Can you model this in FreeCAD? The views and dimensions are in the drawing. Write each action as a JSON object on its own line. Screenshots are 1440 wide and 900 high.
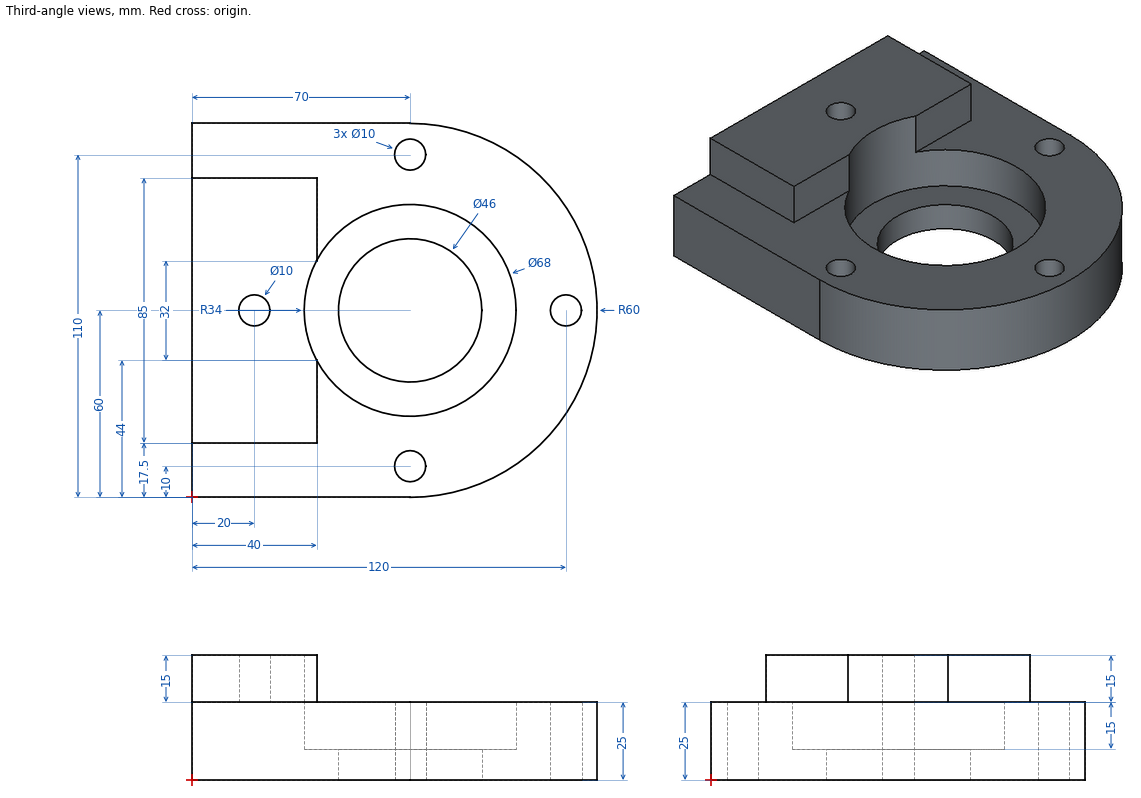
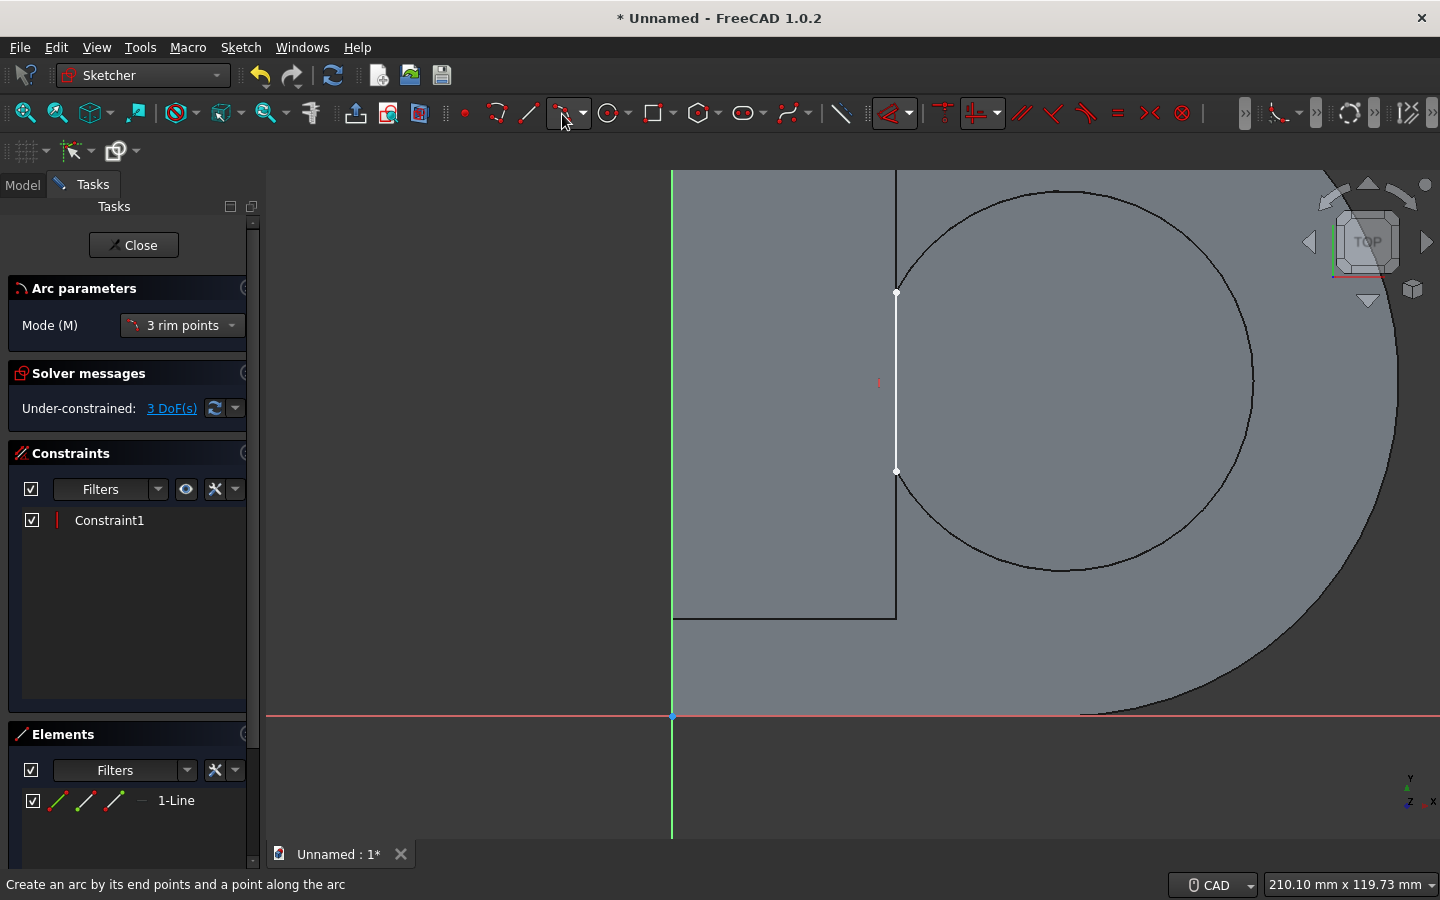
{"action": "left_click", "coordinate": [896, 293]}
{"action": "left_click", "coordinate": [896, 472]}
{"action": "left_click", "coordinate": [874, 381]}
{"action": "key", "text": "Escape"}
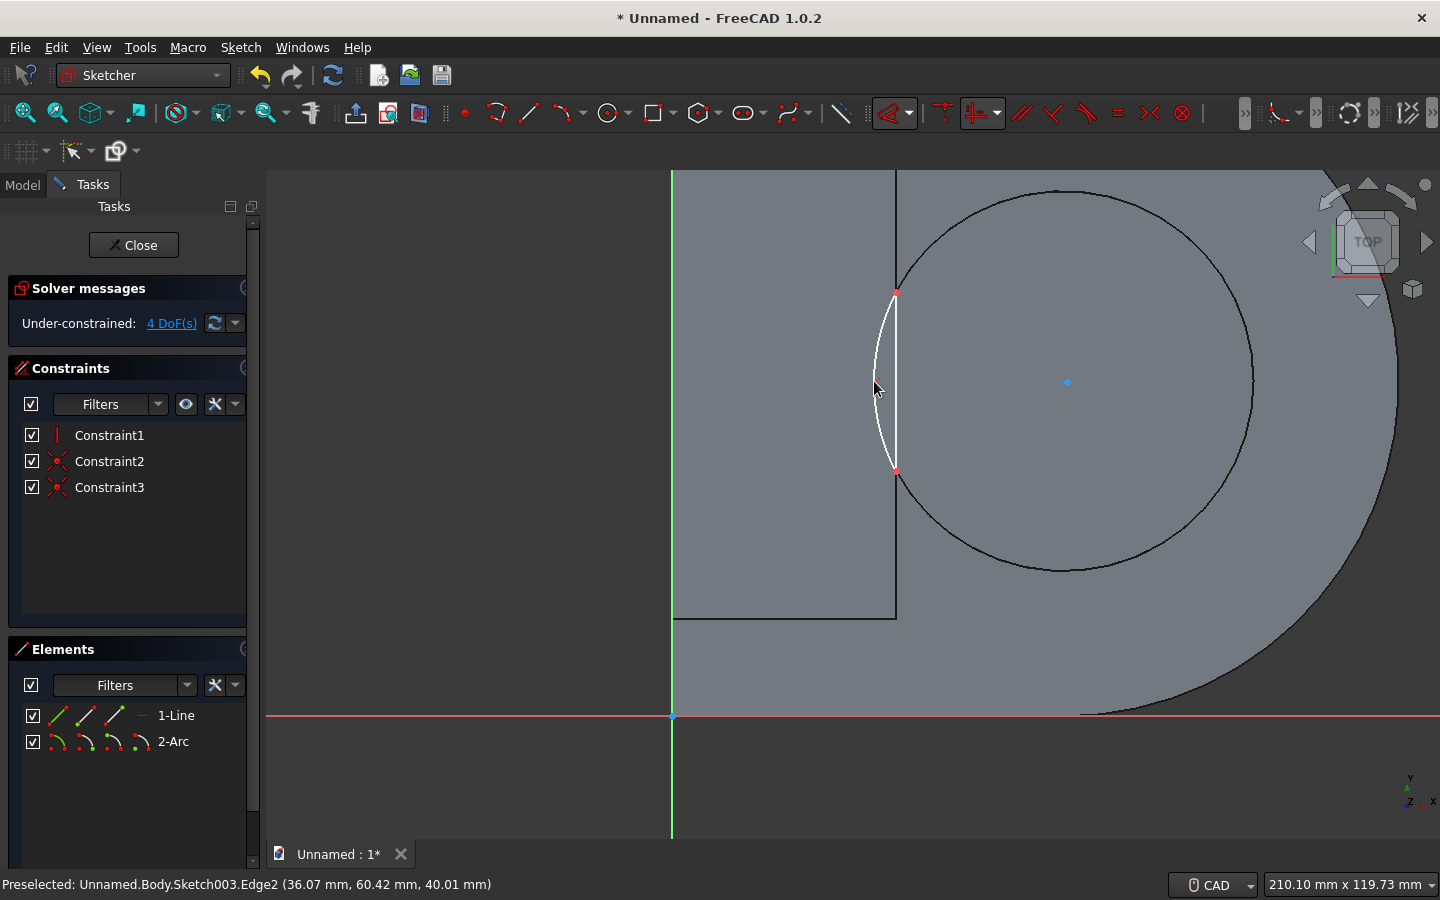
{"action": "left_click", "coordinate": [878, 346]}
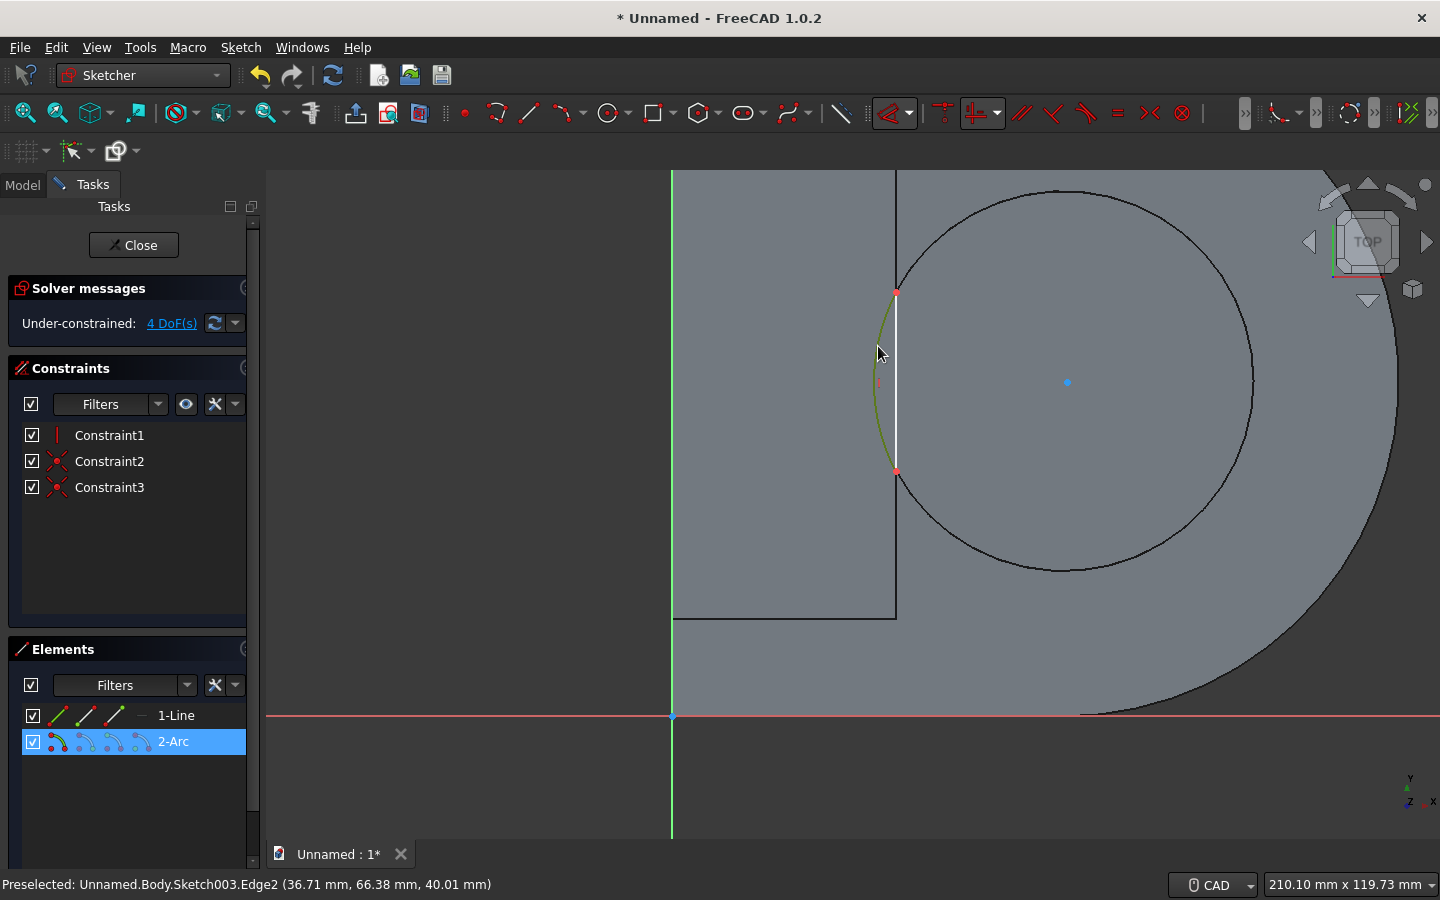
{"action": "left_click", "coordinate": [912, 114]}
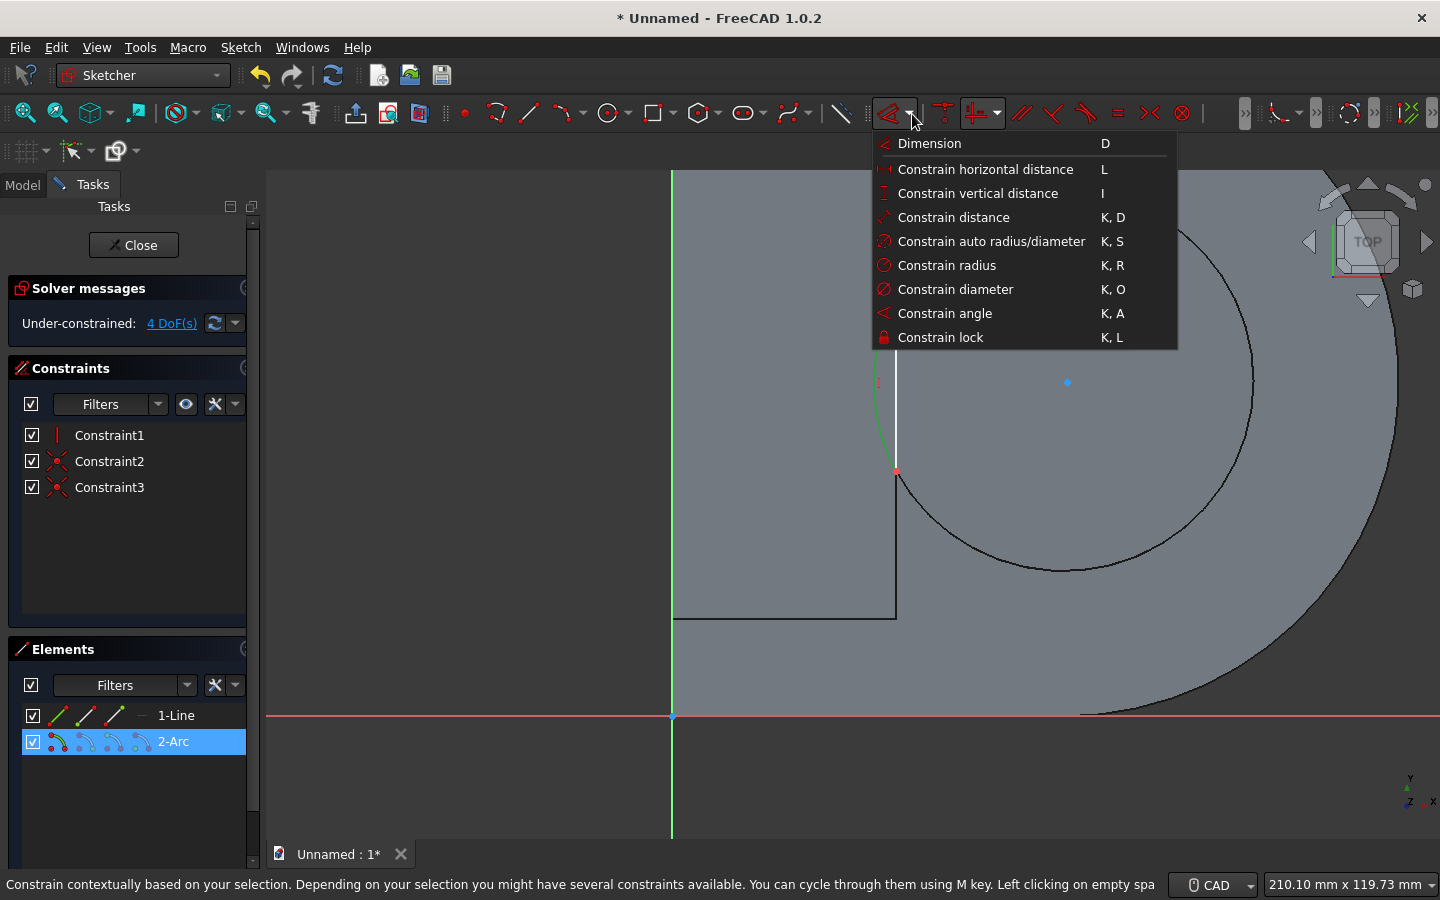
{"action": "left_click", "coordinate": [1025, 265]}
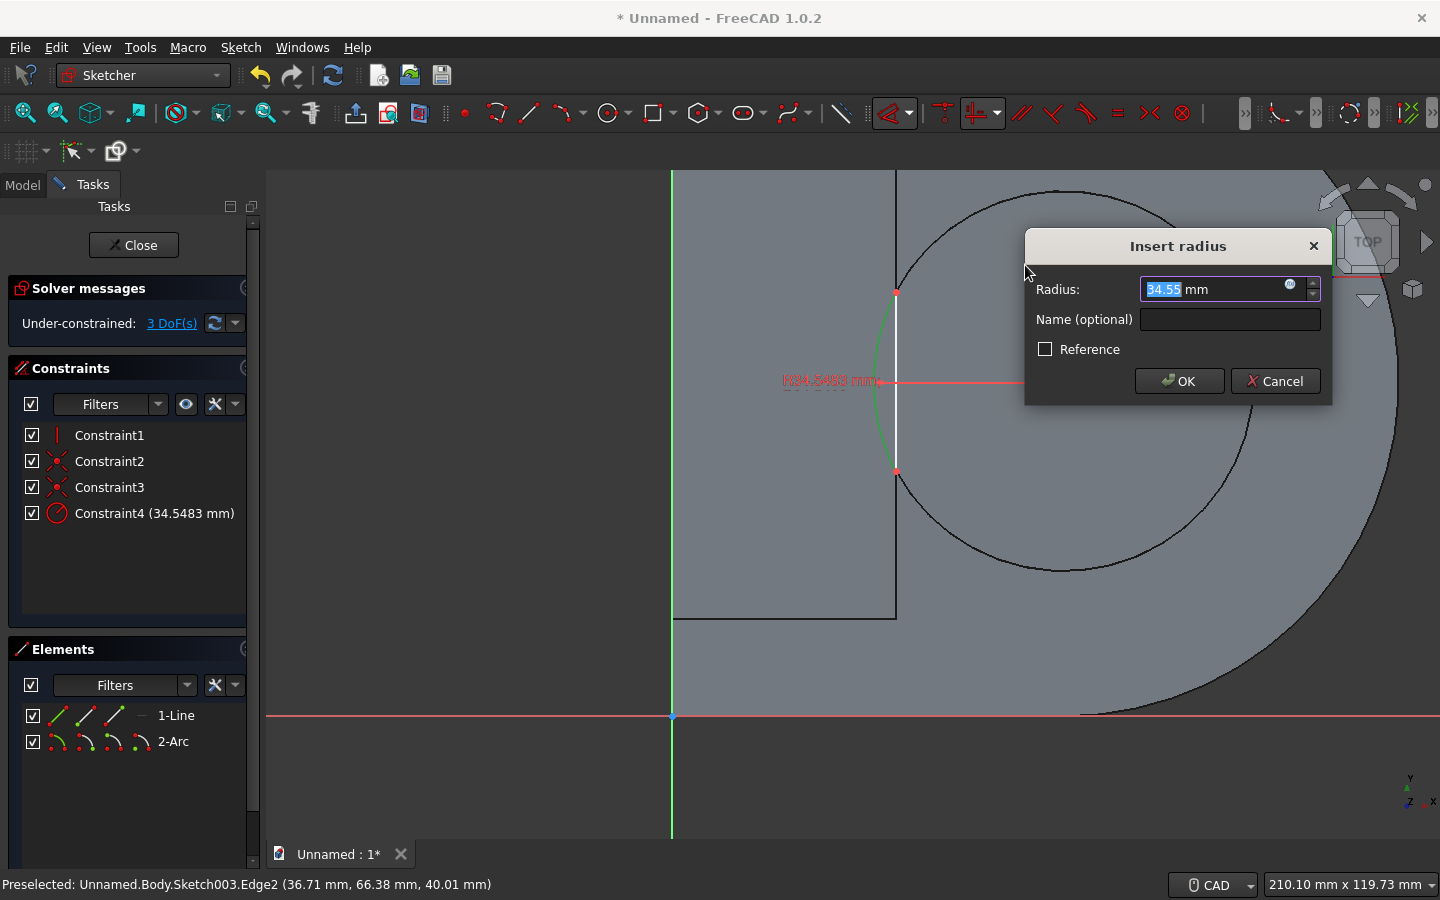
{"action": "type", "text": "34"}
{"action": "key", "text": "Return"}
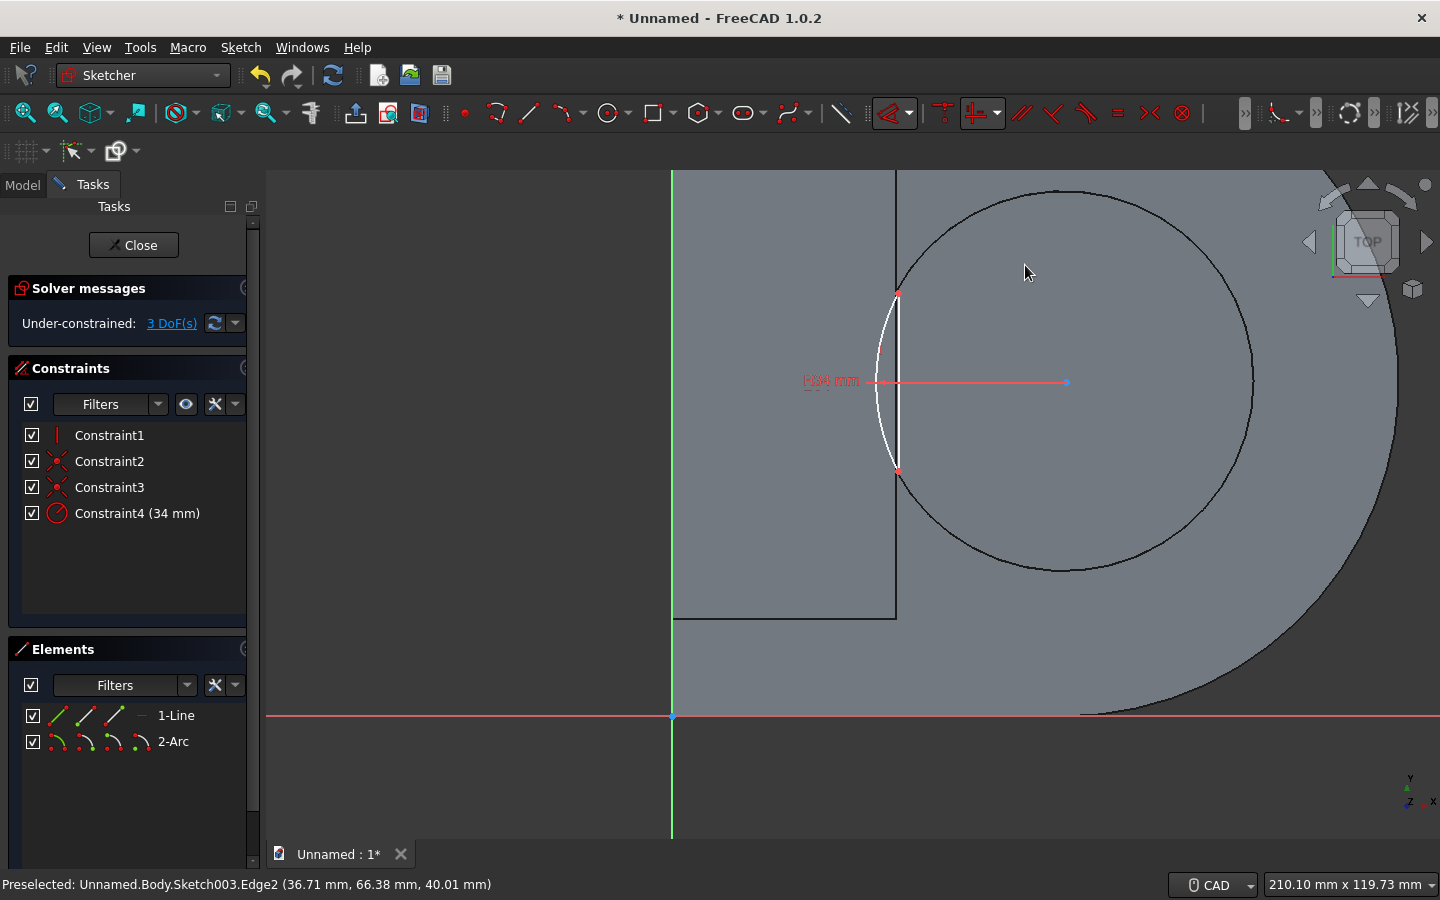
{"action": "left_click", "coordinate": [899, 418]}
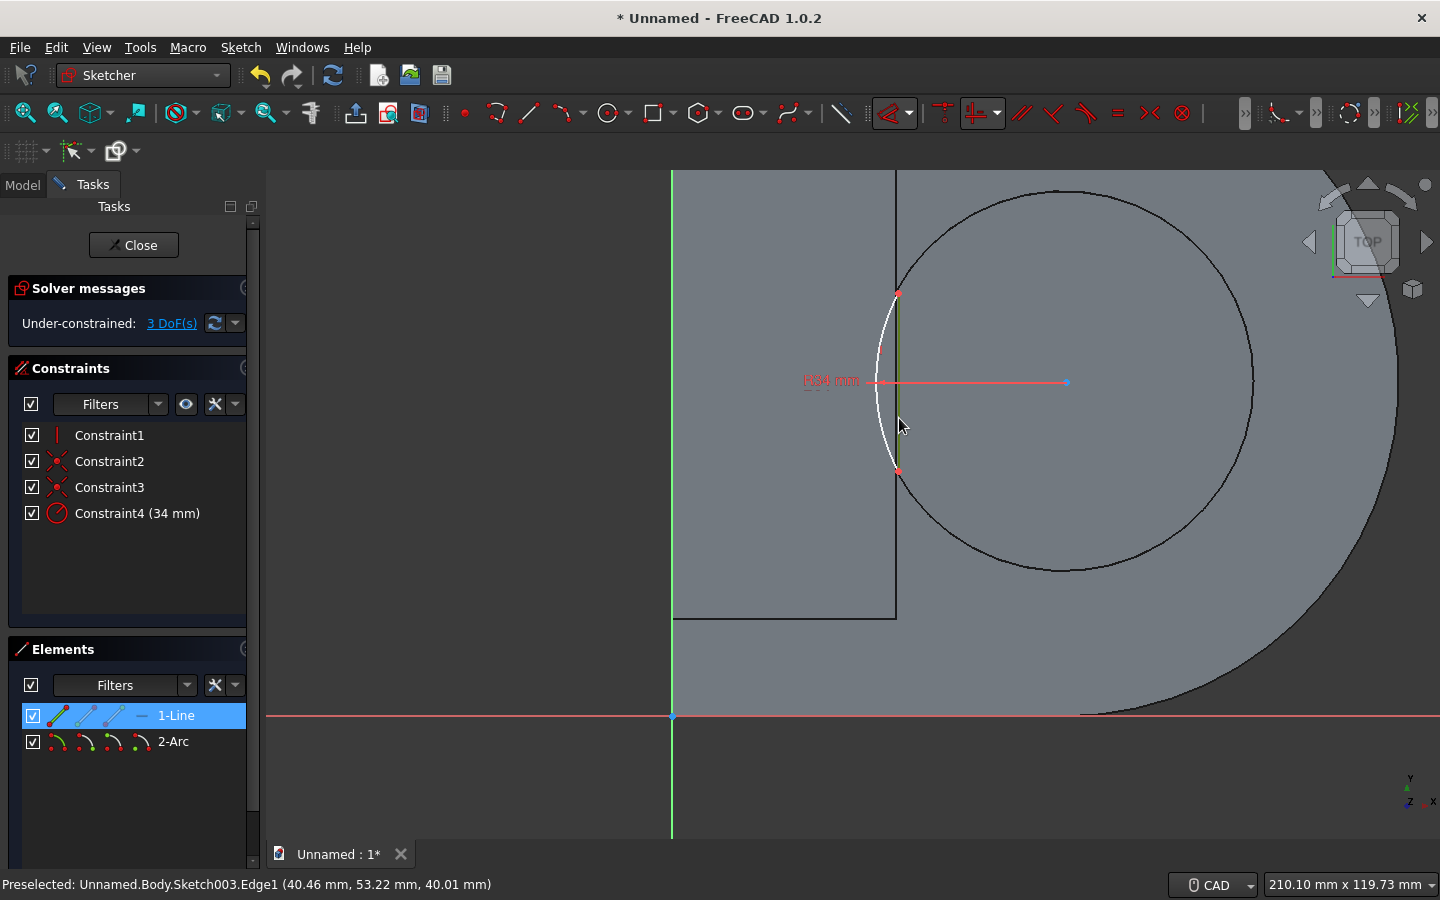
{"action": "key", "text": "i"}